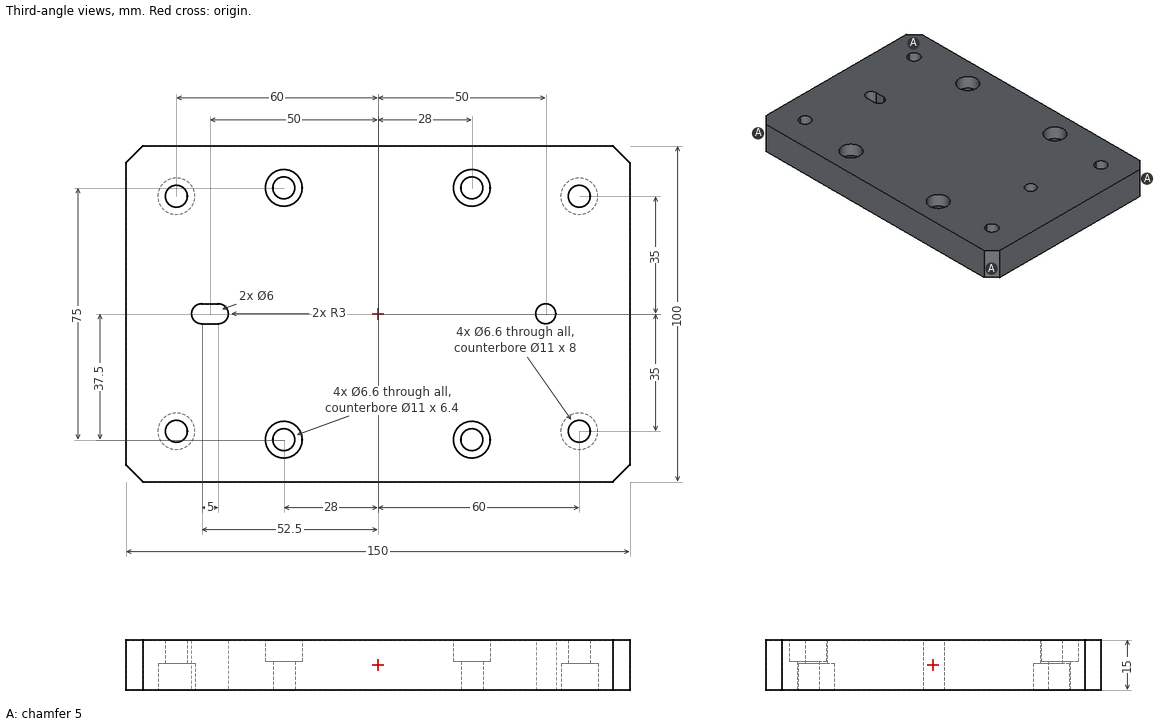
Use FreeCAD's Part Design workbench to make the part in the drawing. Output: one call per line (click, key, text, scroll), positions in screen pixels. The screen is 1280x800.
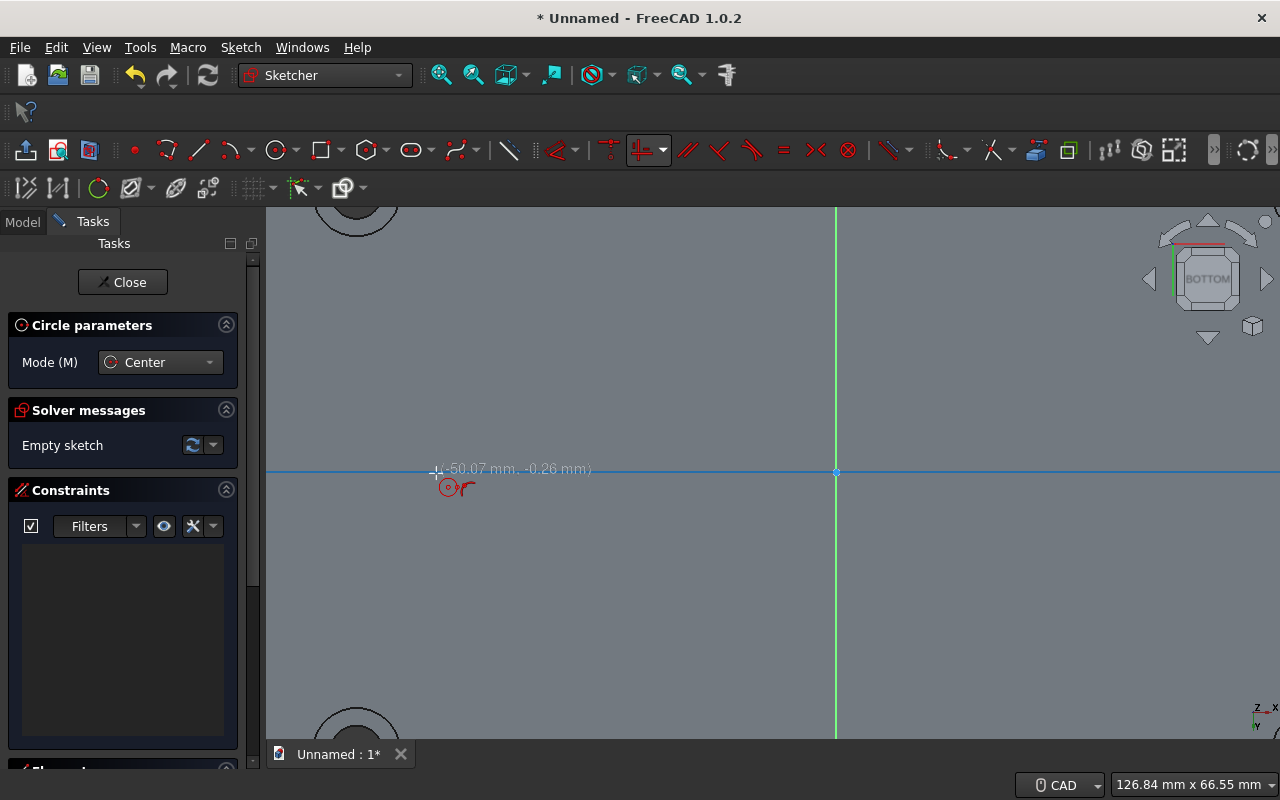
click(436, 472)
move(453, 455)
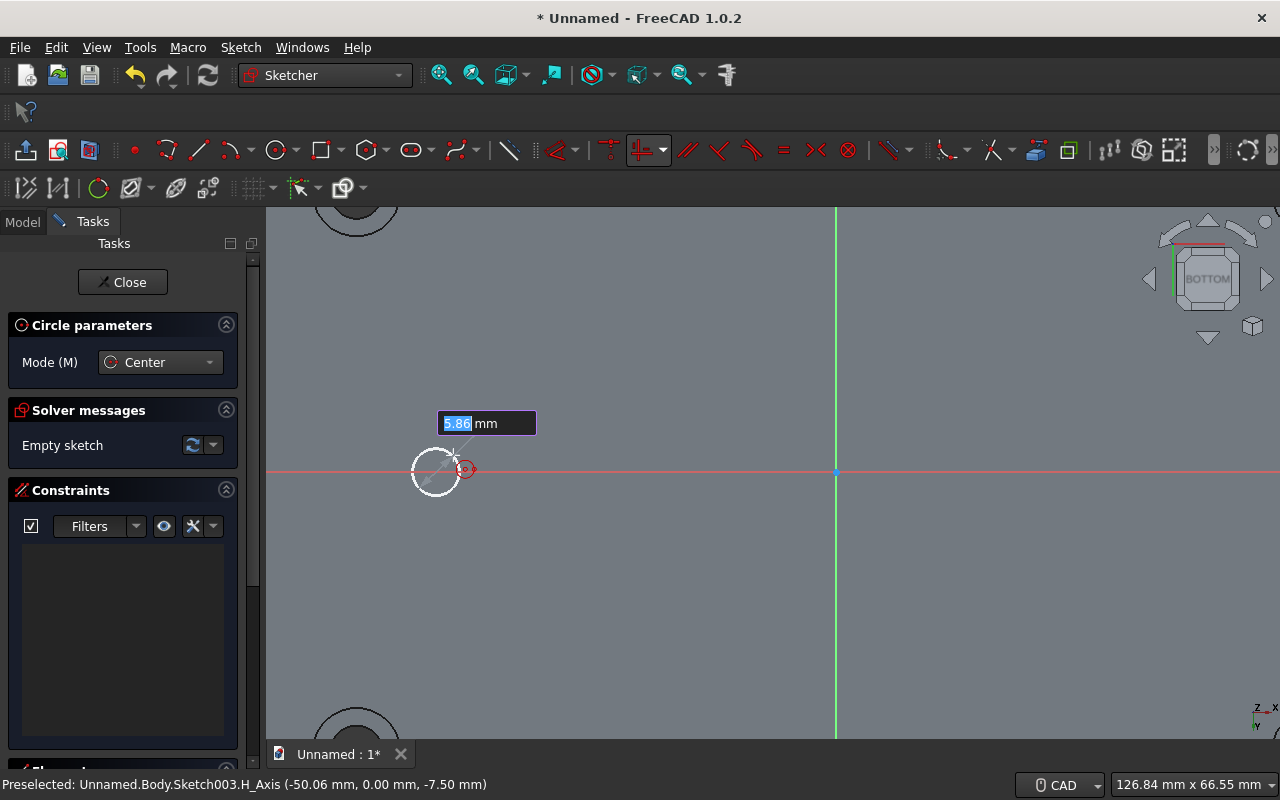
text(6)
key(Return)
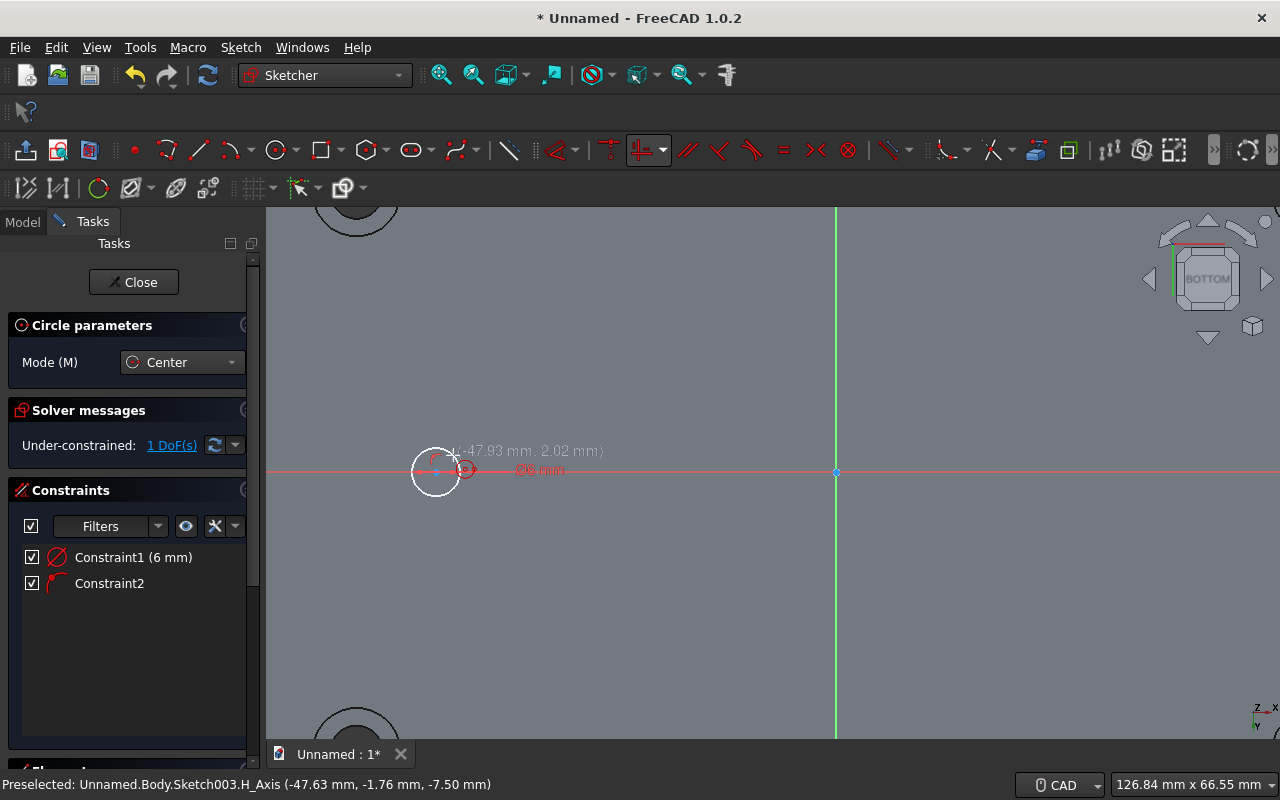
scroll(437, 475, down, 2)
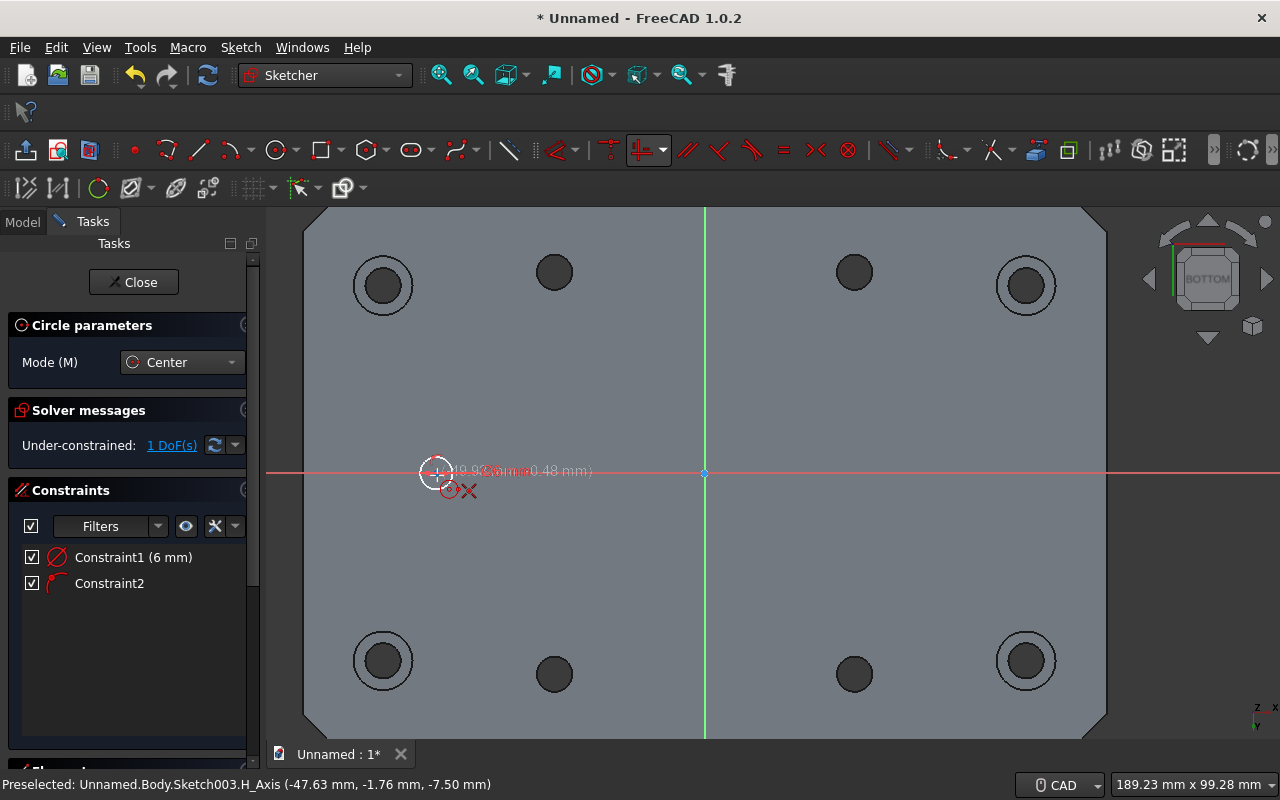
scroll(973, 473, up, 2)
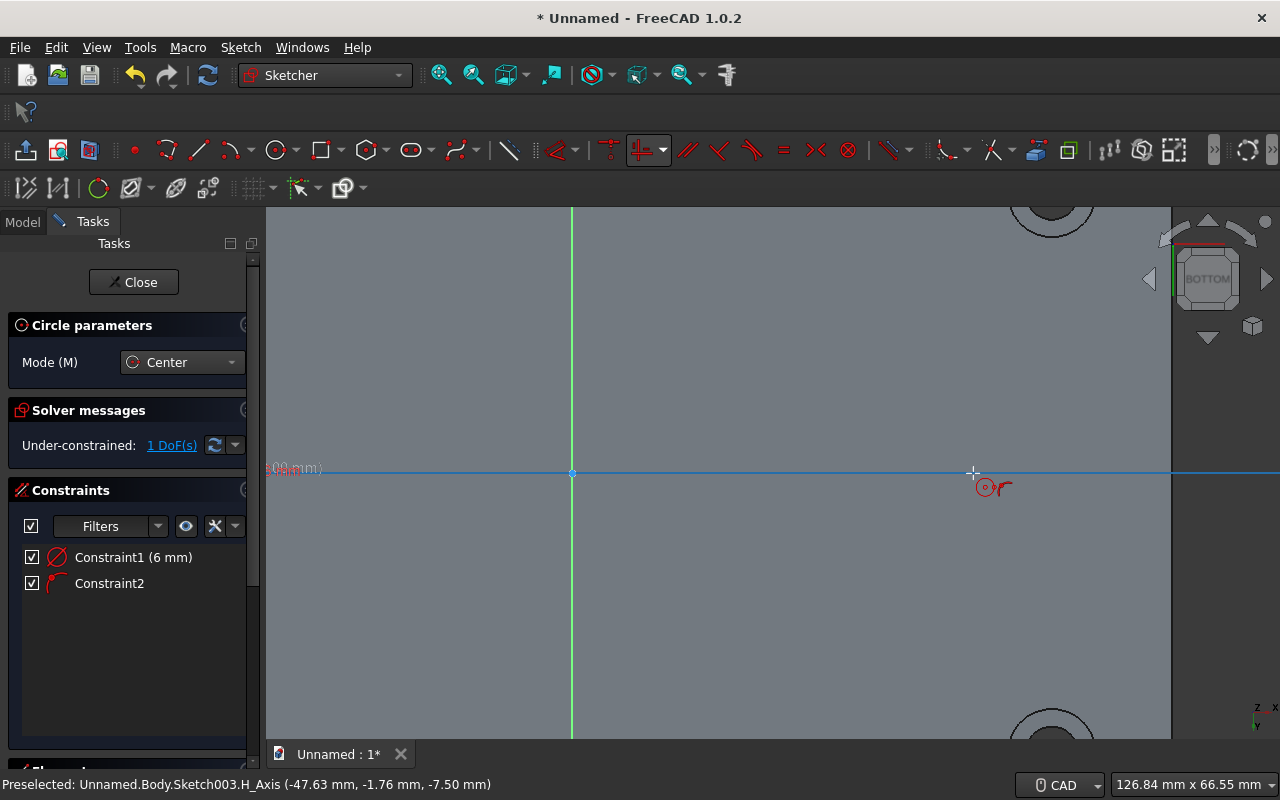
click(972, 473)
move(989, 456)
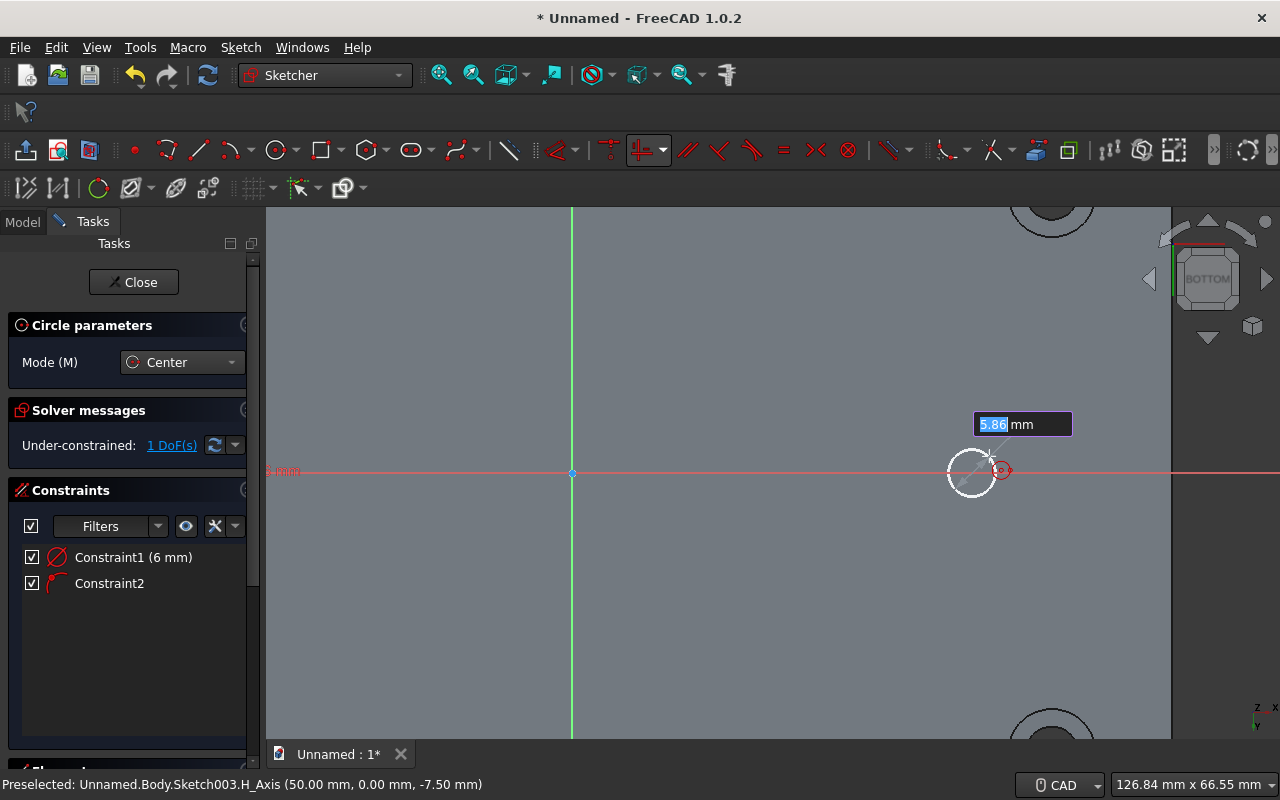
text(6)
key(Return)
key(Escape)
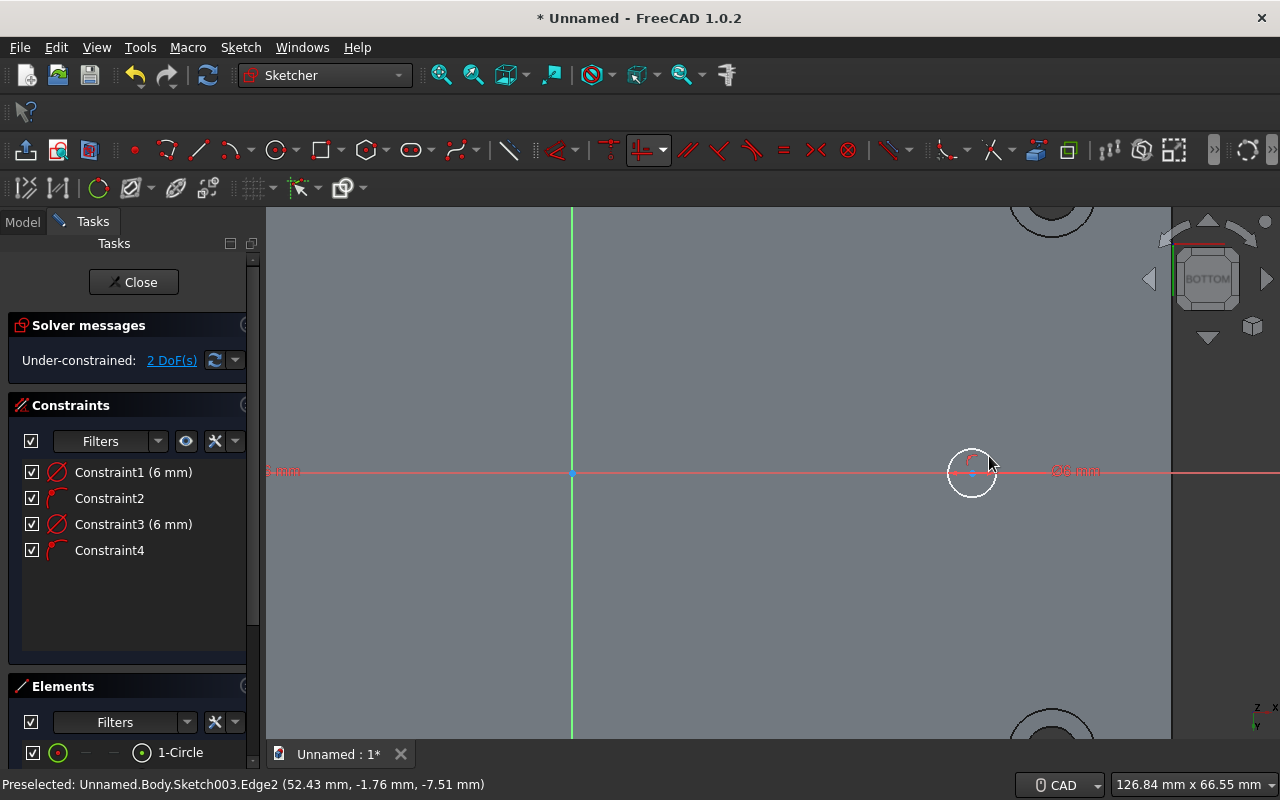
click(556, 150)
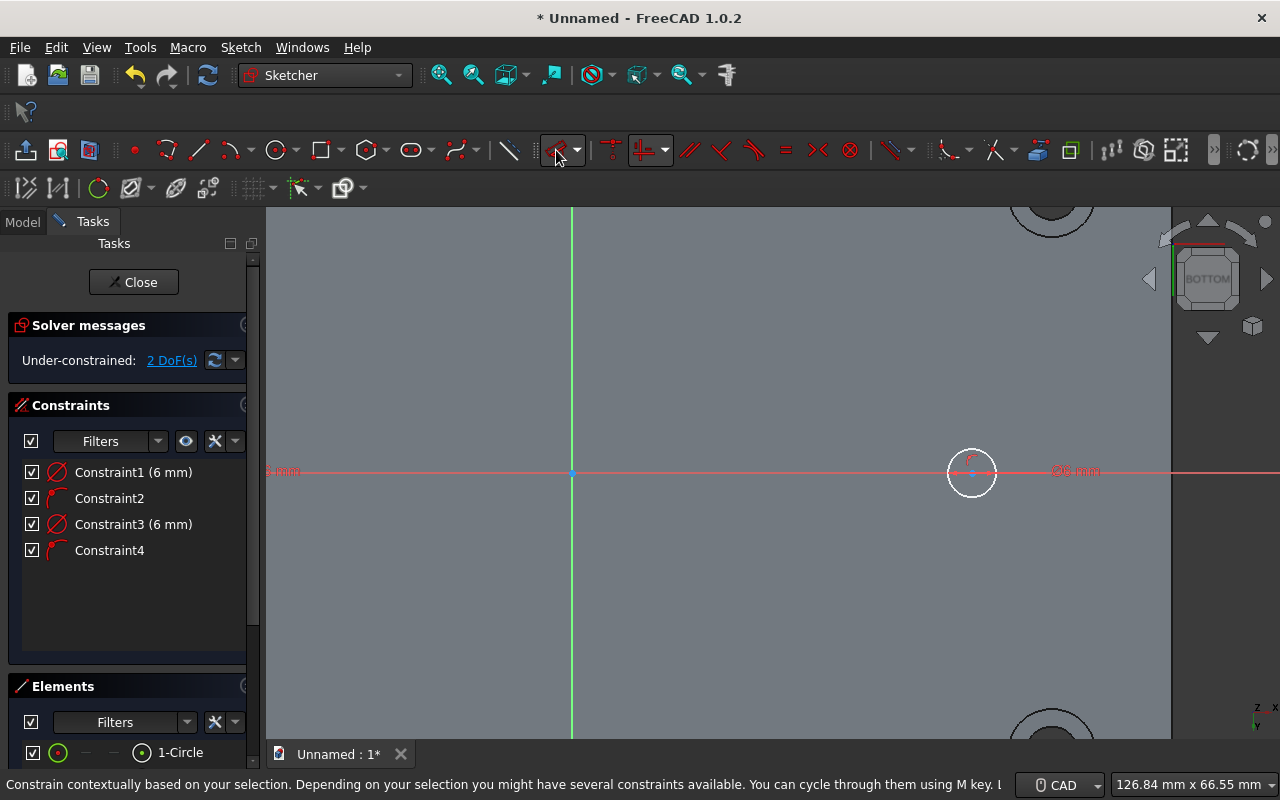
scroll(973, 473, down, 2)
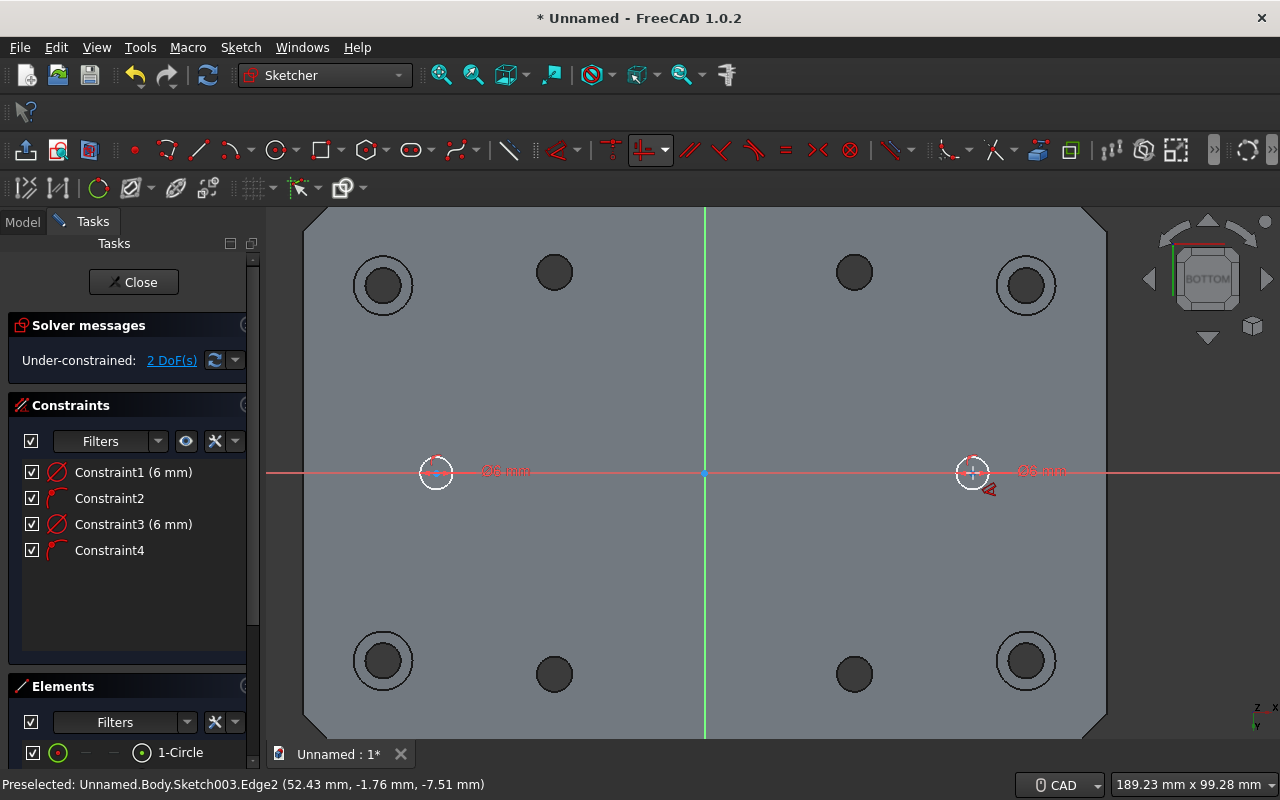
click(436, 473)
click(571, 507)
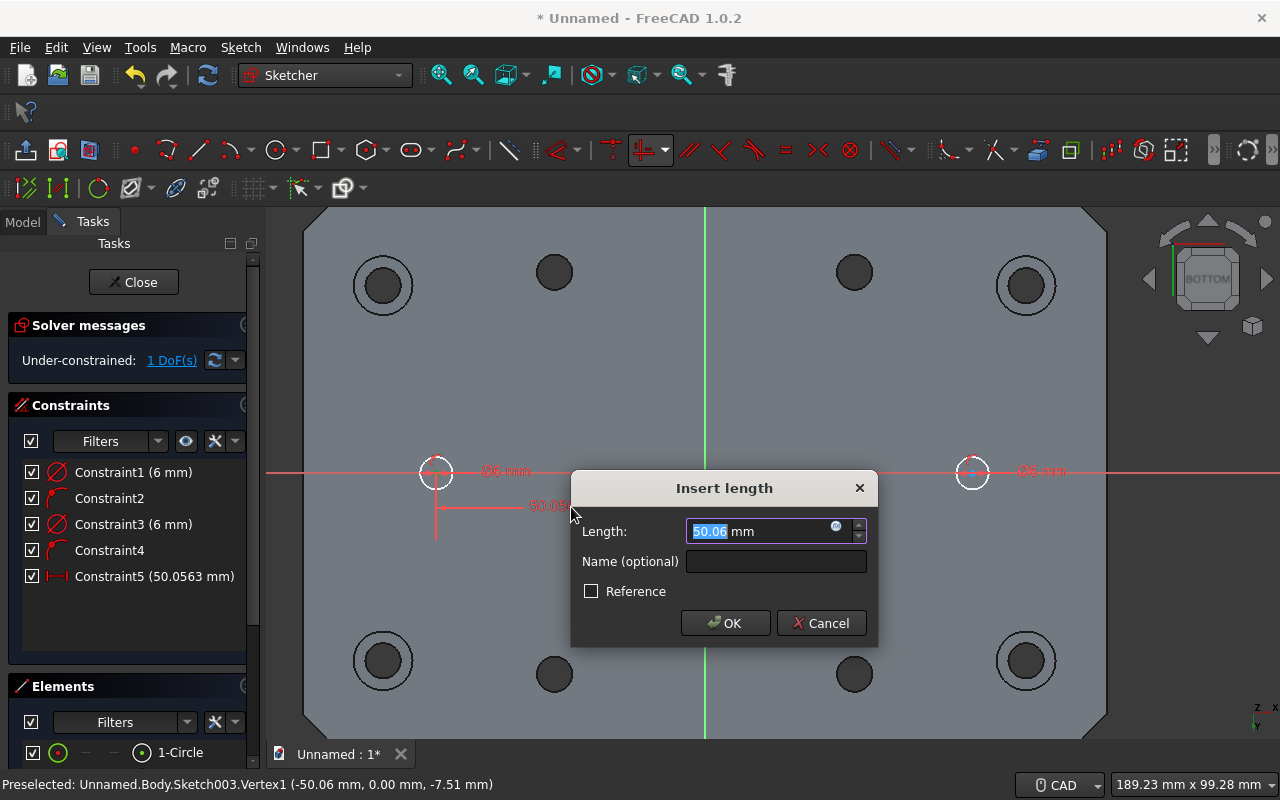
text(50)
key(Return)